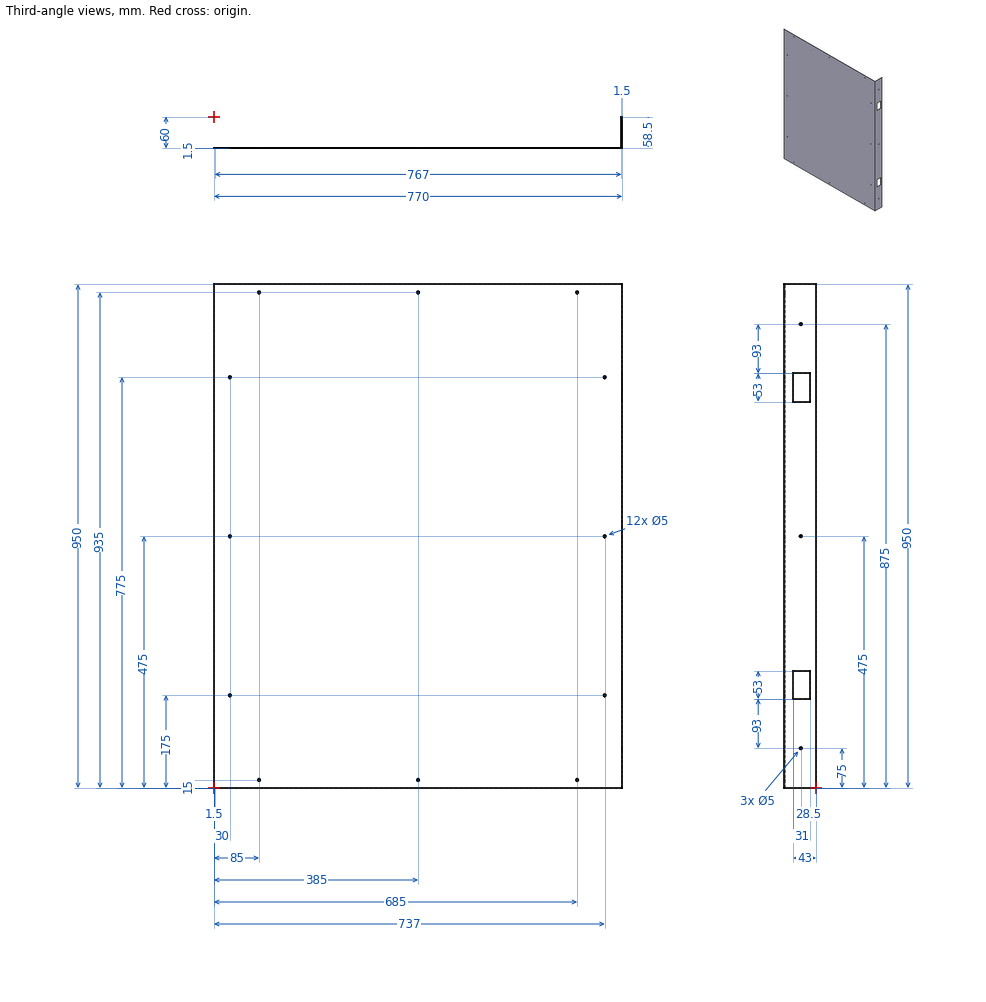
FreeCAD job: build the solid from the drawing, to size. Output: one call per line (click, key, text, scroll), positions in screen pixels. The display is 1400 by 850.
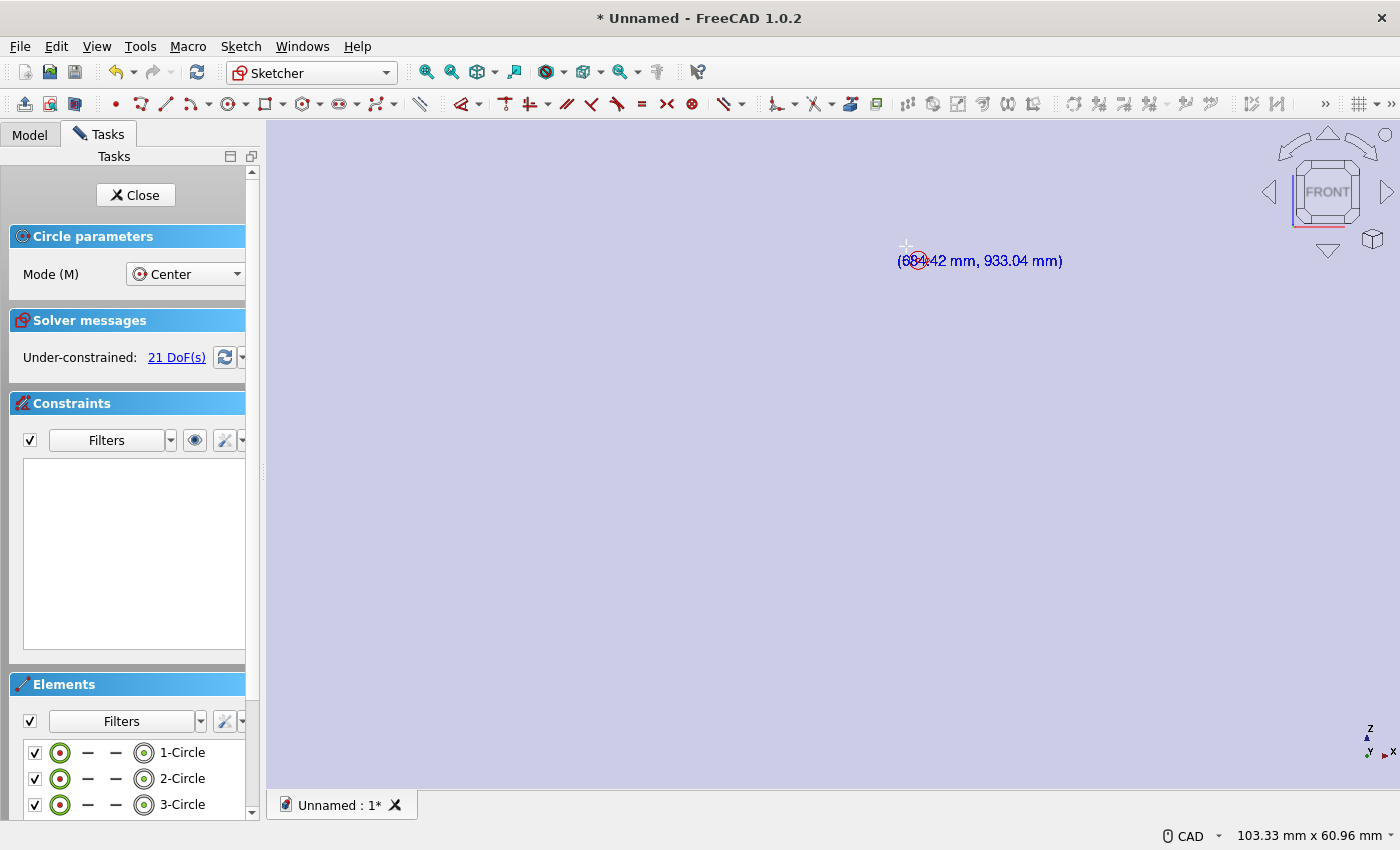
scroll(939, 197, down, 15)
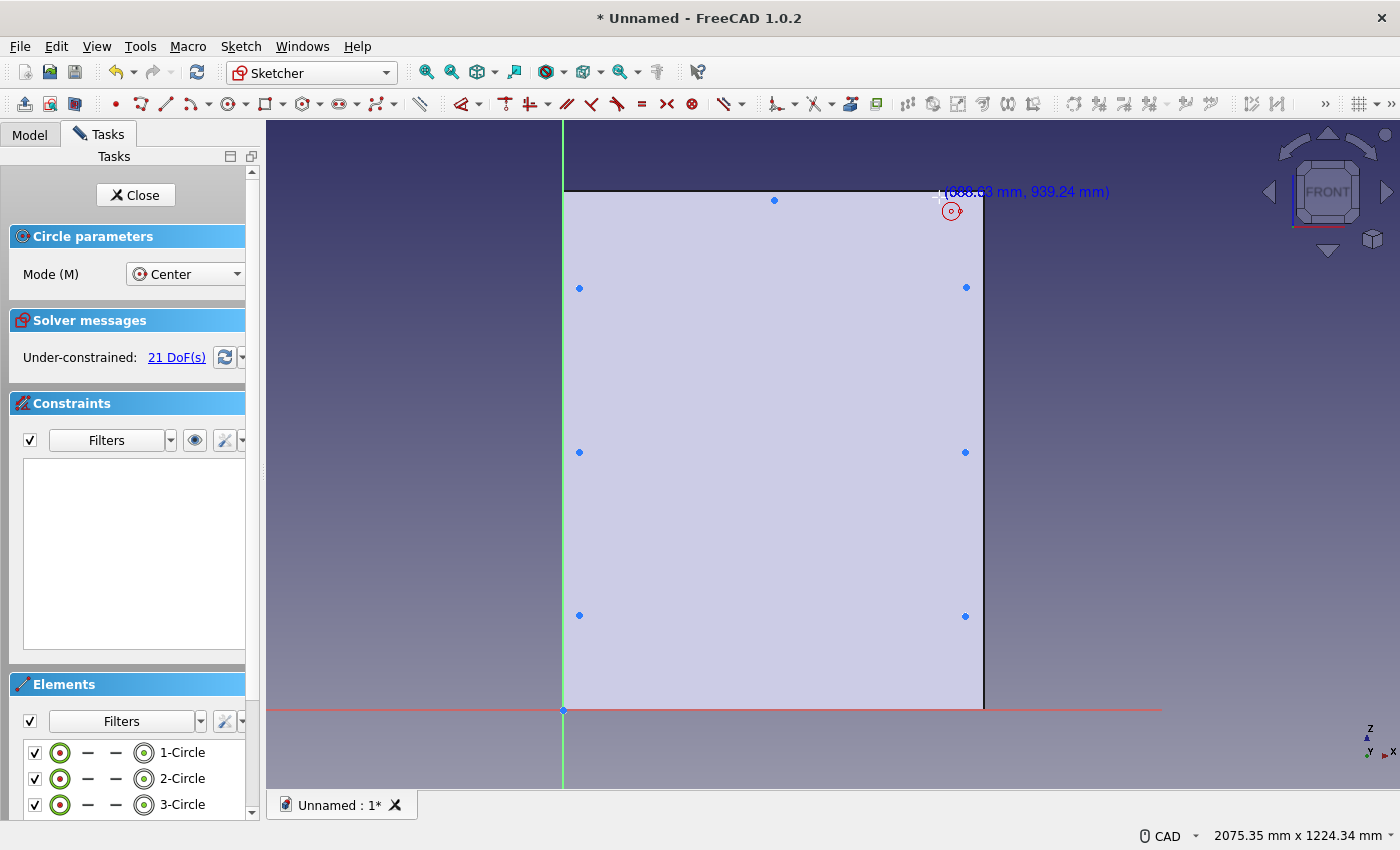
click(938, 199)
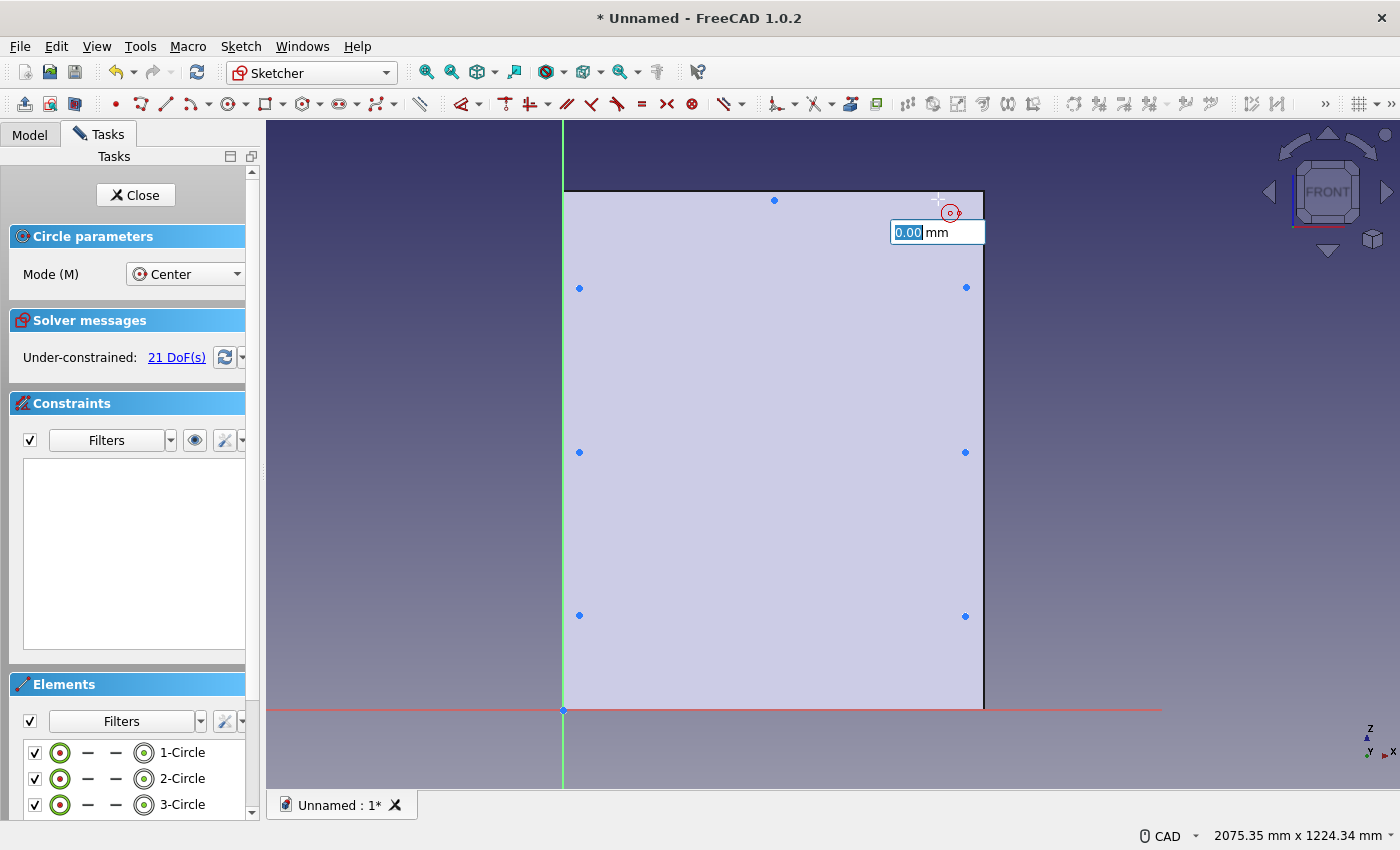
scroll(939, 199, up, 13)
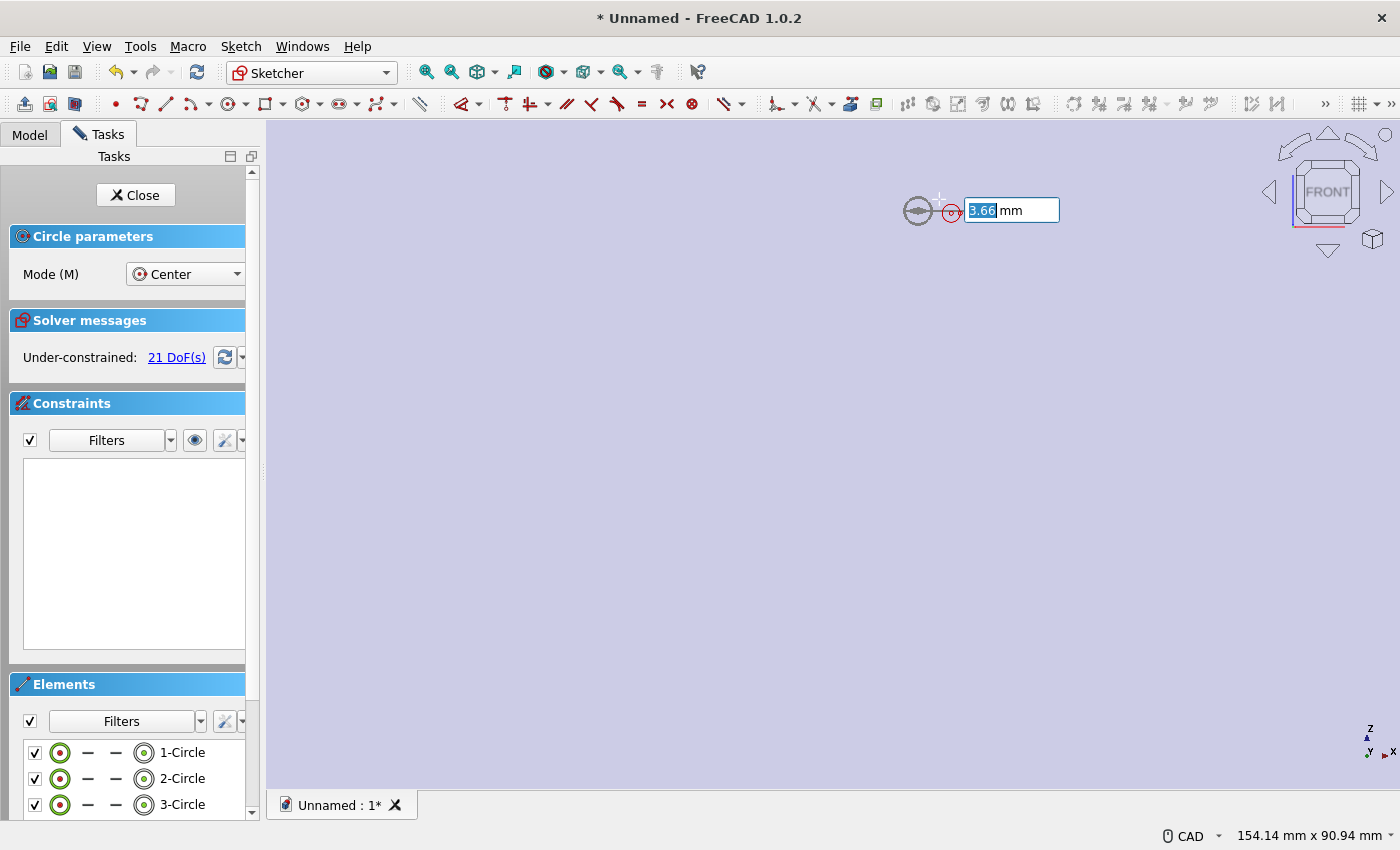
click(925, 191)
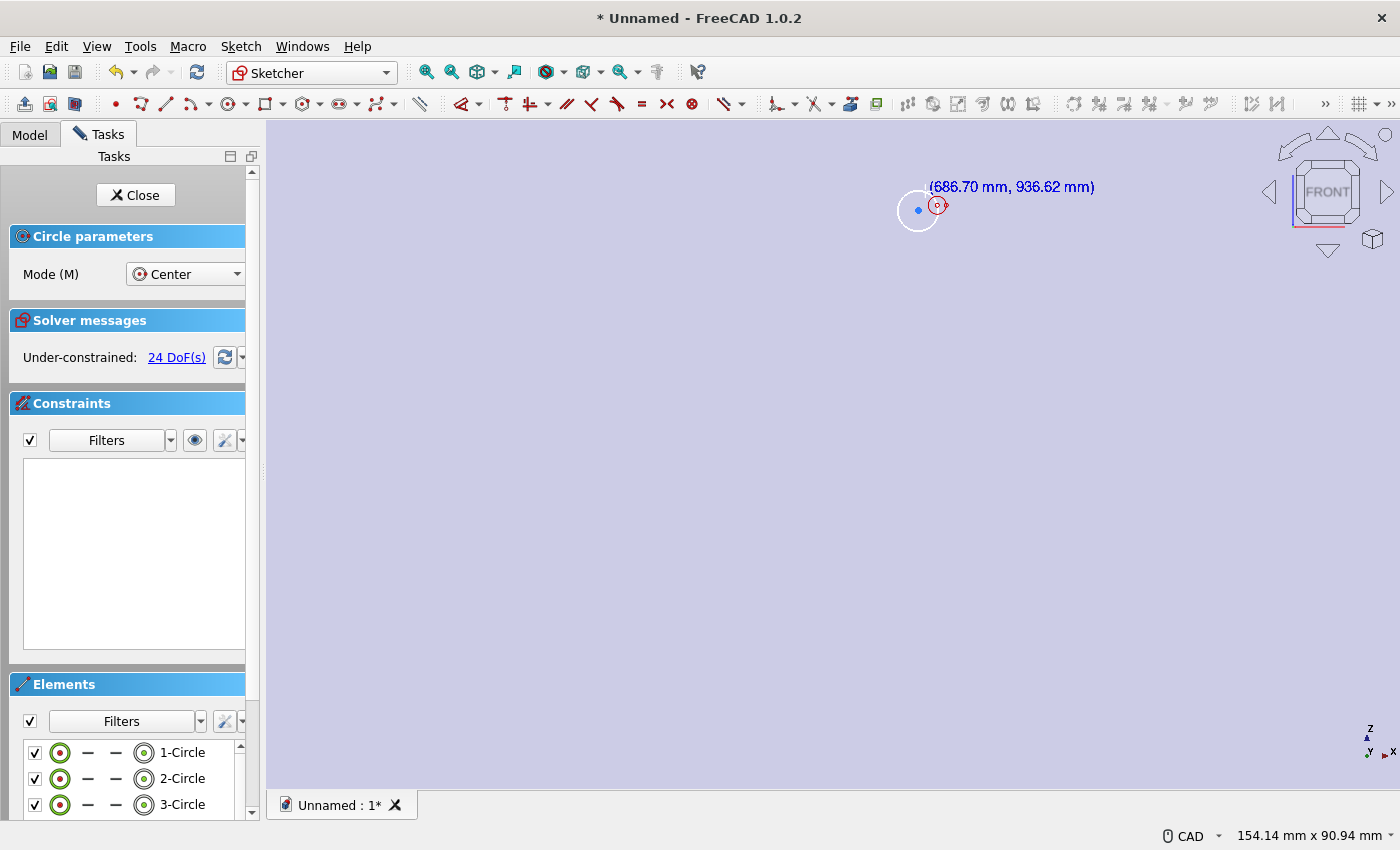
scroll(905, 249, down, 14)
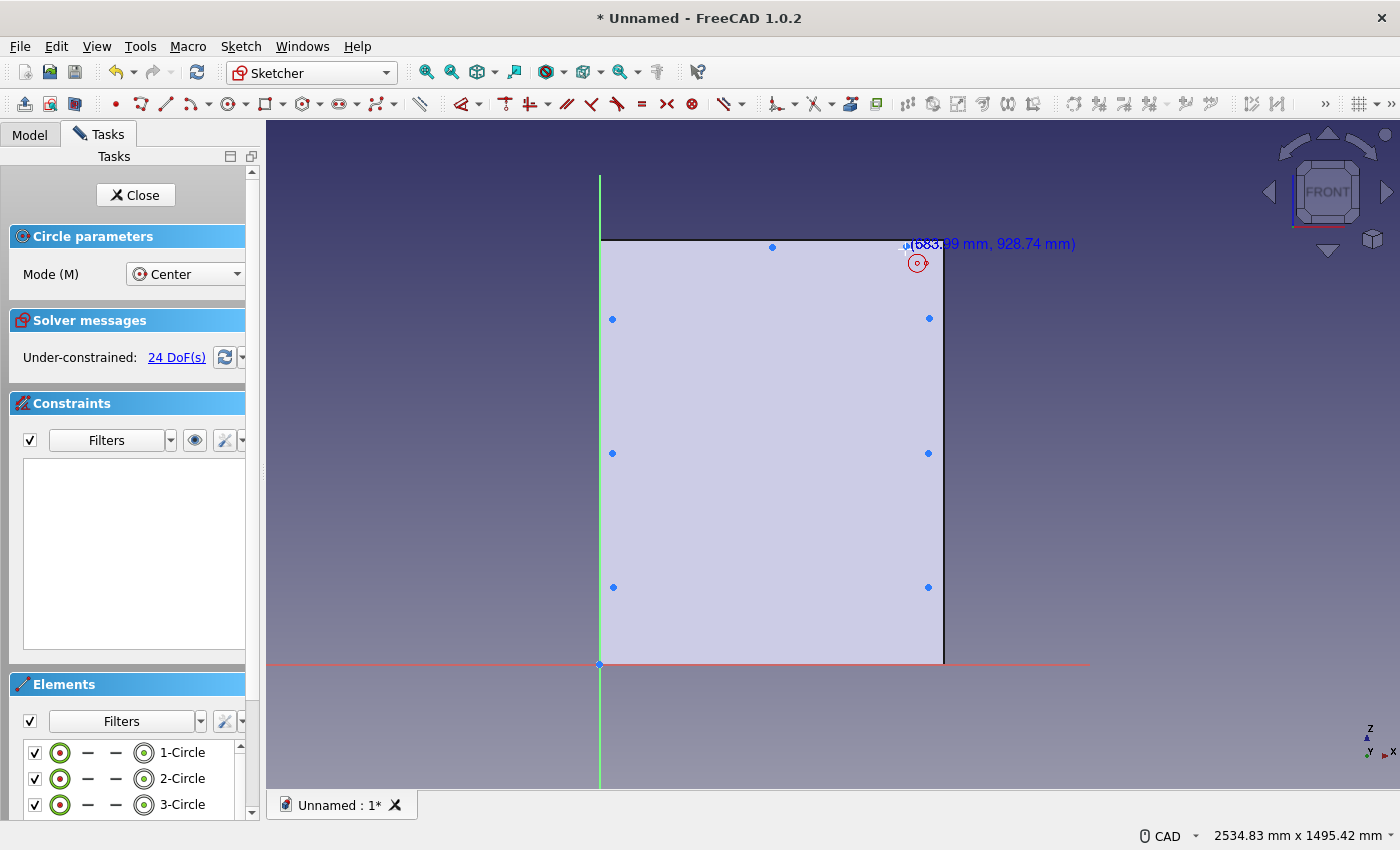
scroll(638, 246, up, 16)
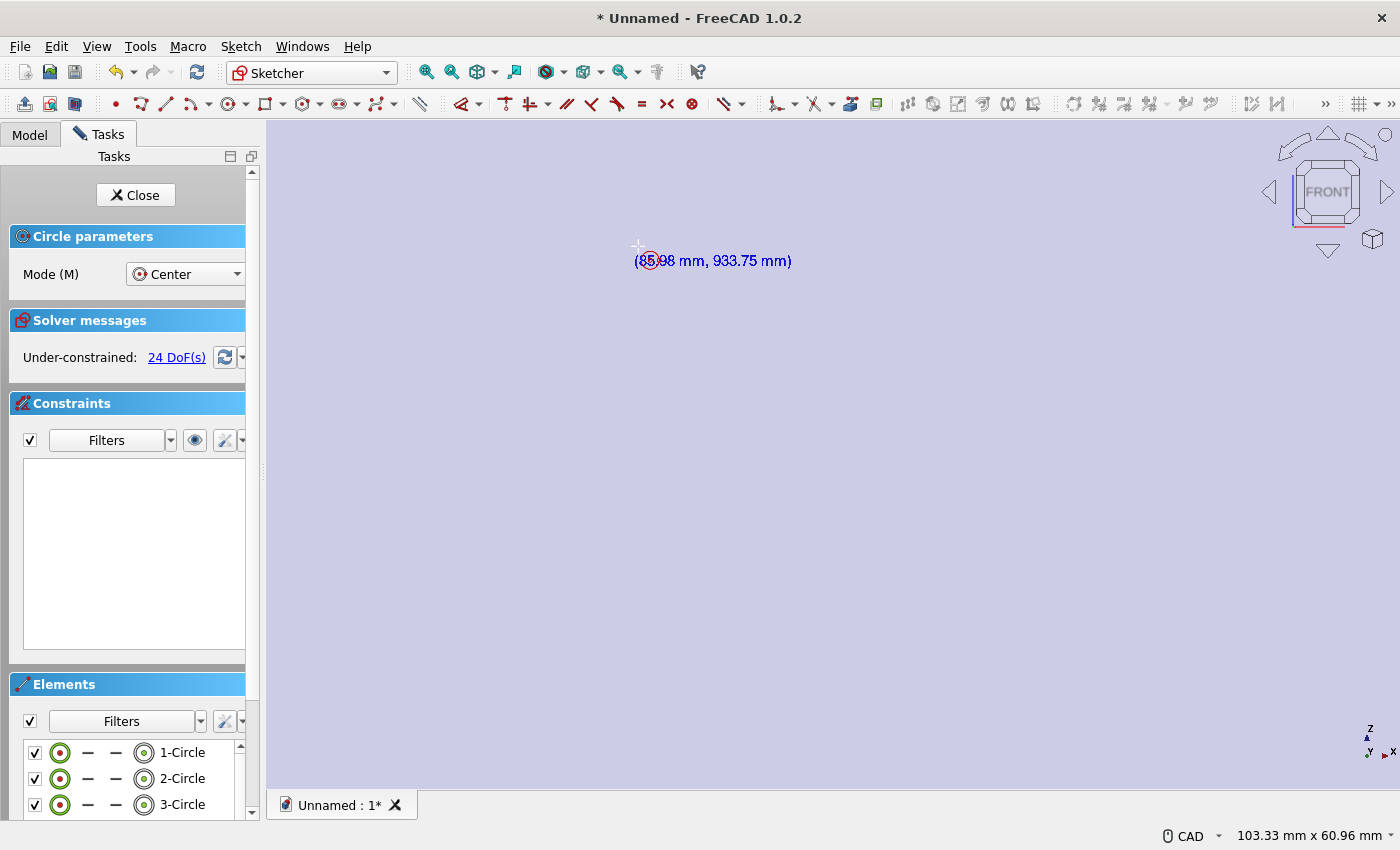
scroll(608, 197, down, 15)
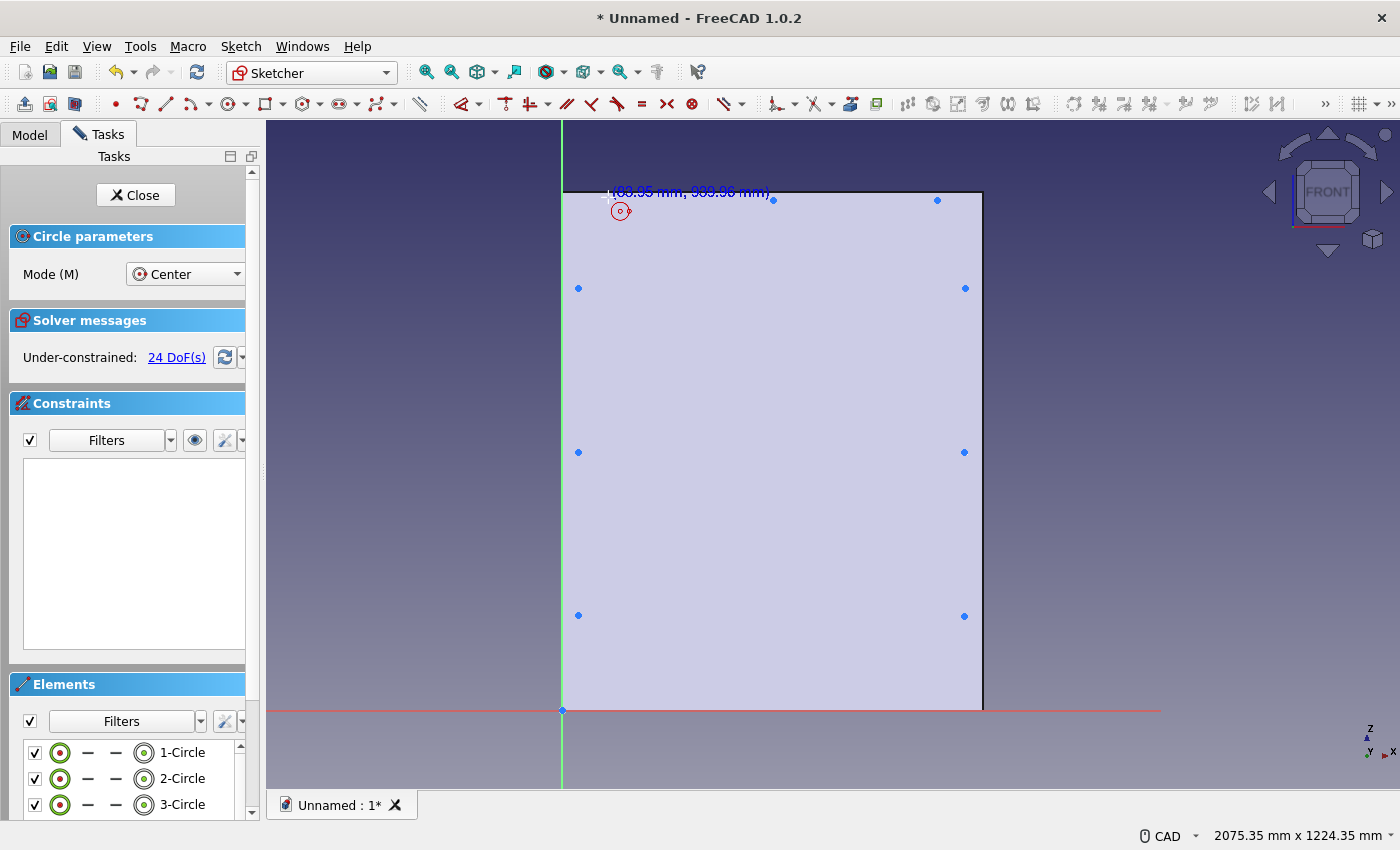
click(609, 200)